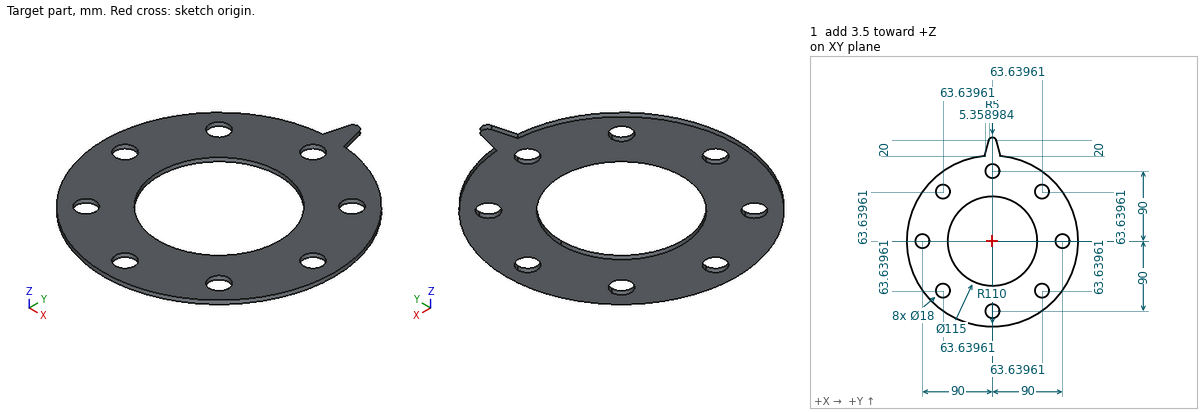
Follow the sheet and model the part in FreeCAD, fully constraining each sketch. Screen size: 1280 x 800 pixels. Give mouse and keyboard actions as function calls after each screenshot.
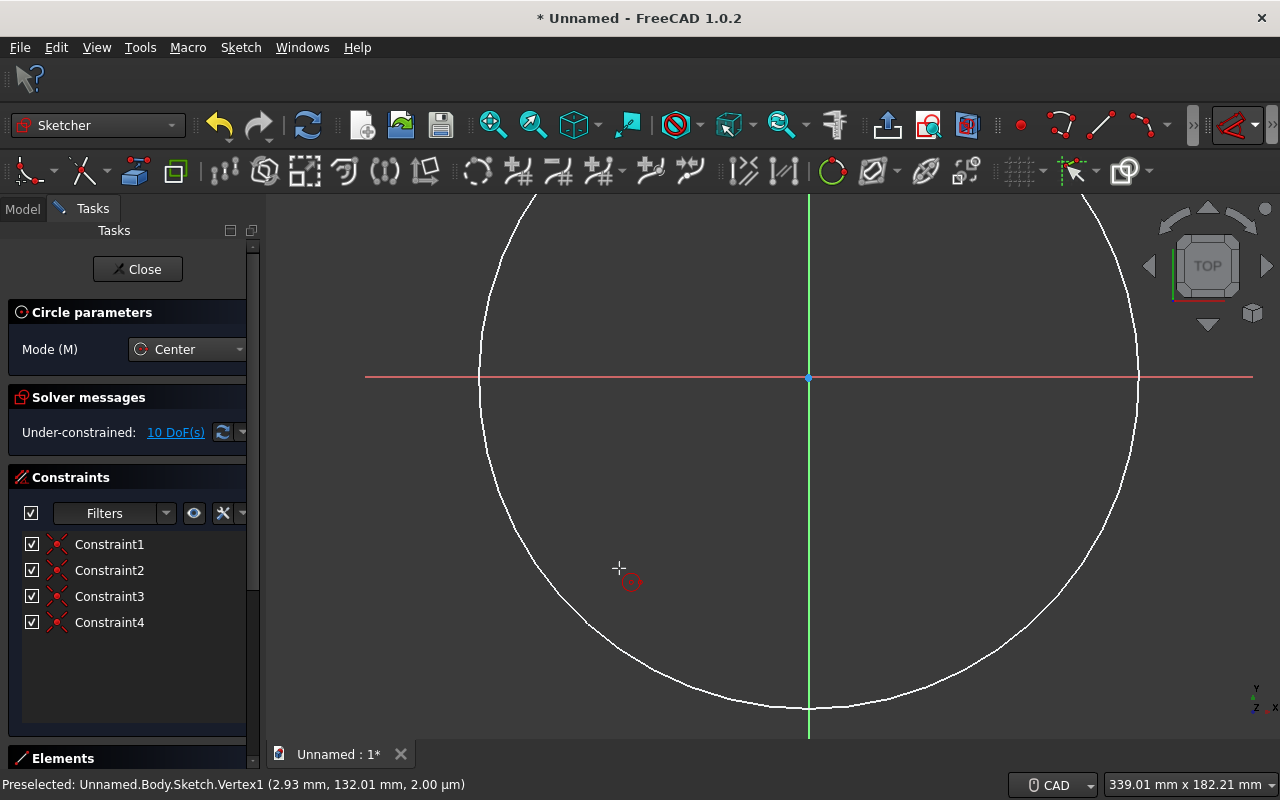
click(619, 567)
click(638, 548)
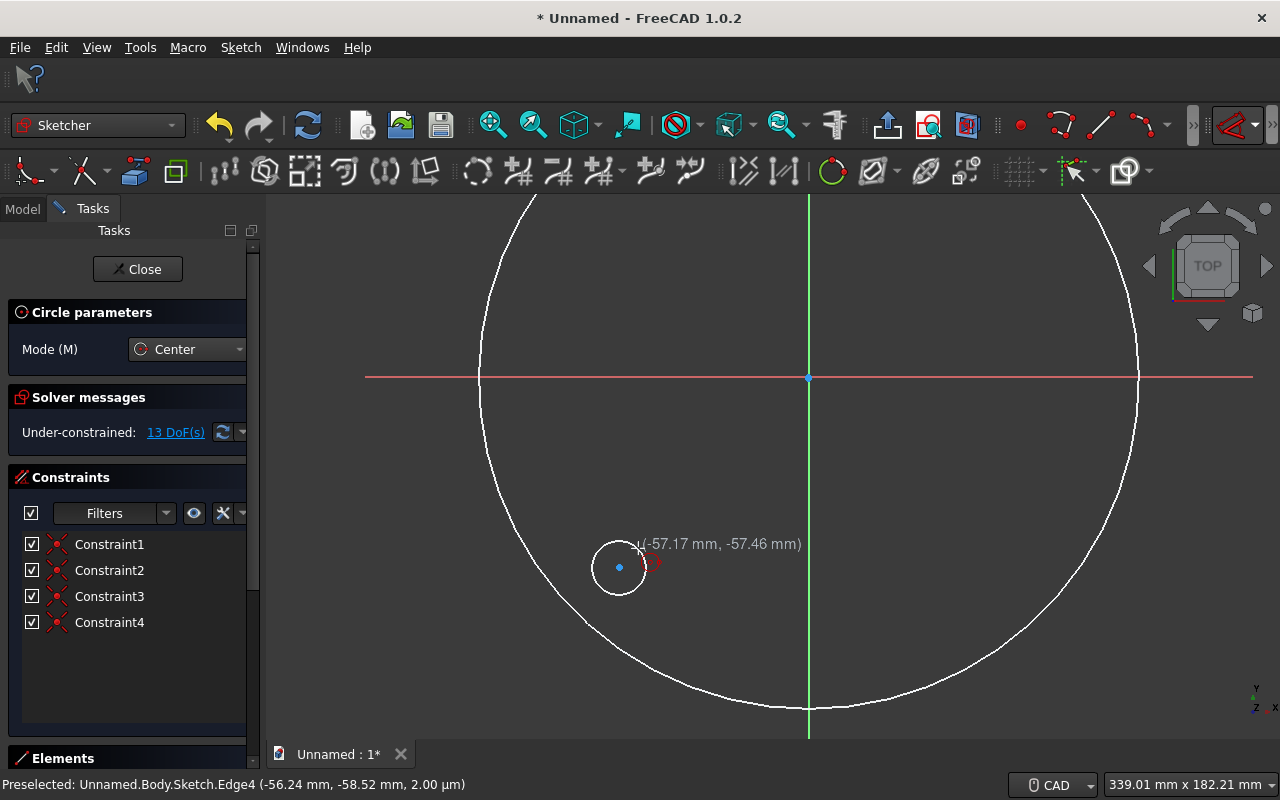
click(809, 646)
click(828, 627)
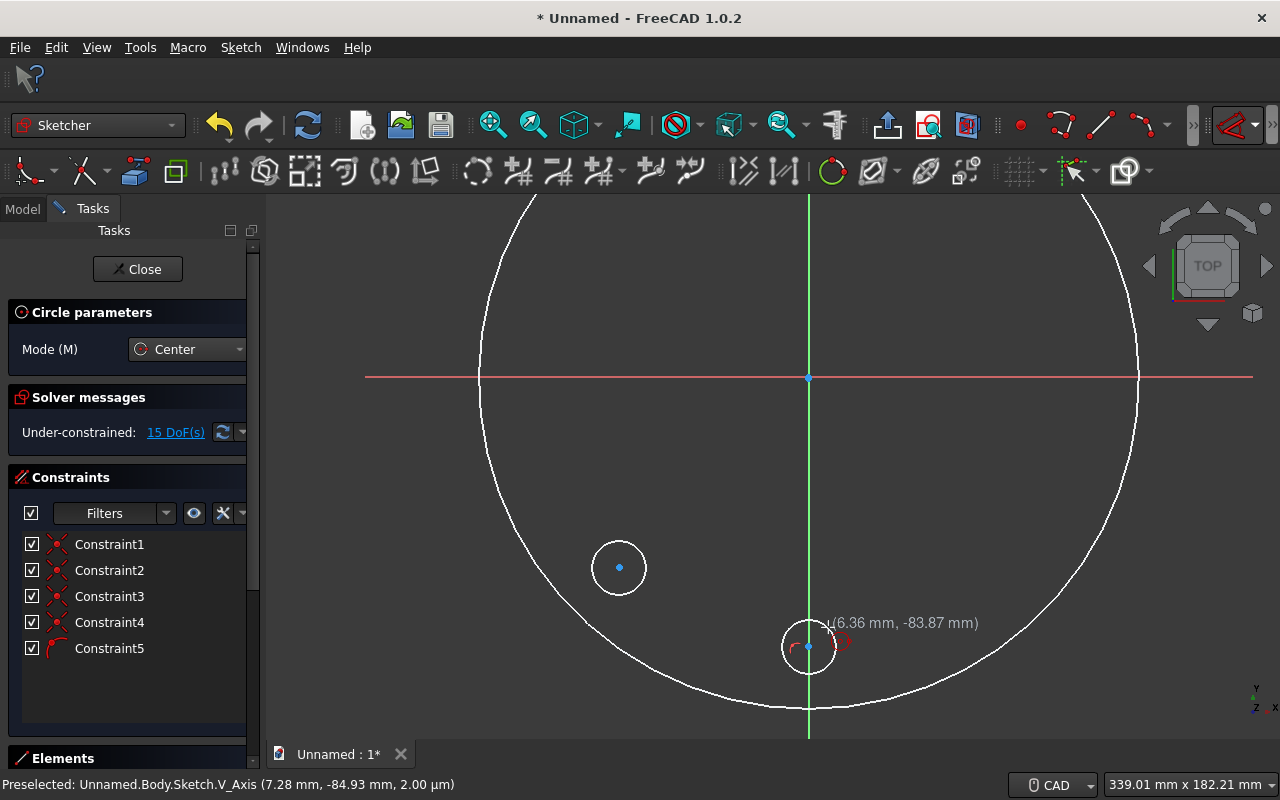
click(999, 567)
click(1018, 548)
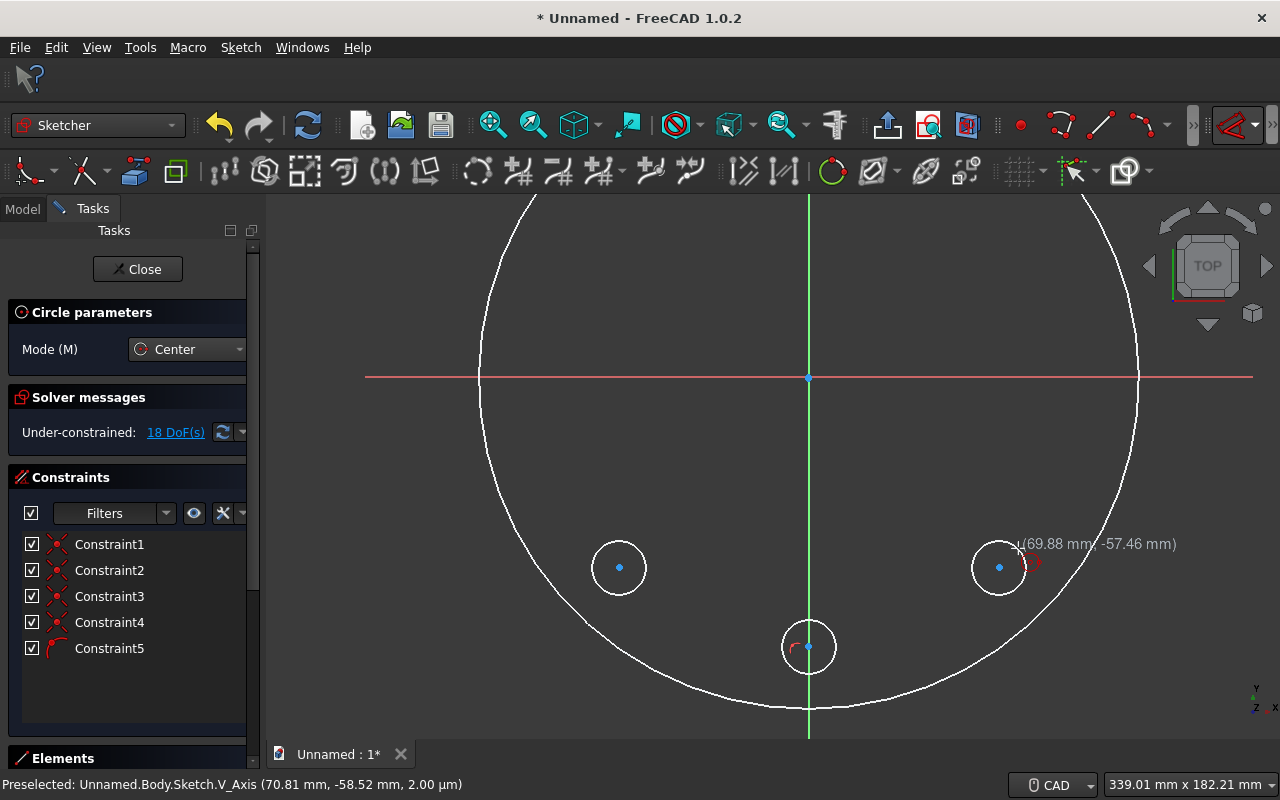
click(540, 377)
click(559, 358)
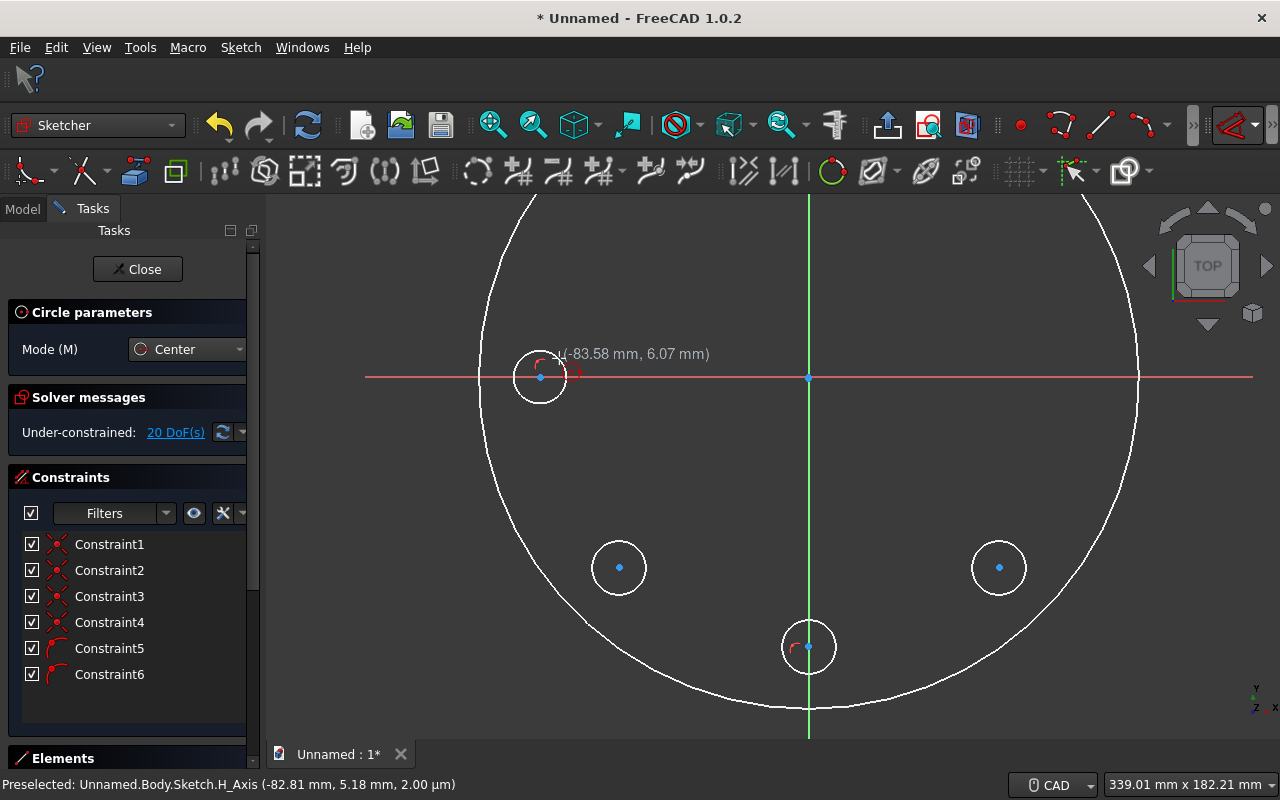
scroll(619, 568, down, 4)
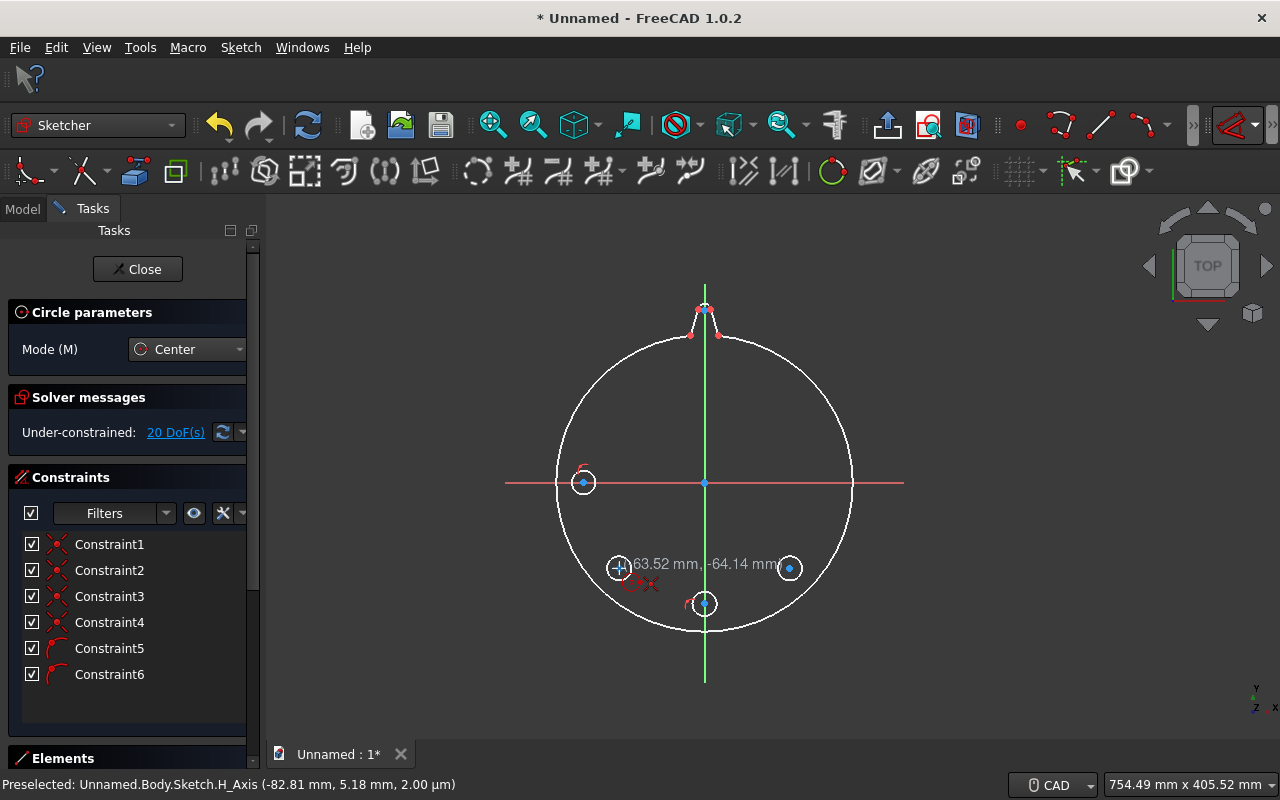
scroll(619, 397, up, 4)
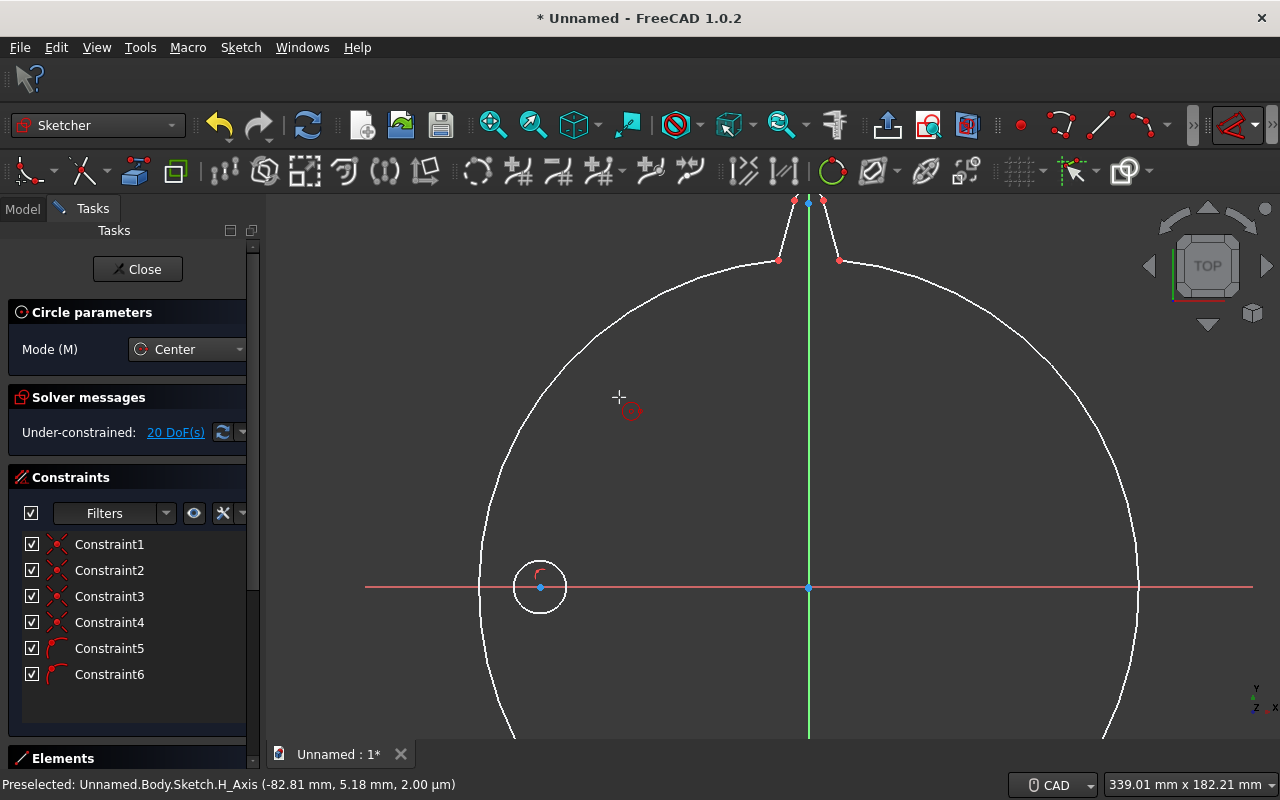
click(619, 397)
click(638, 378)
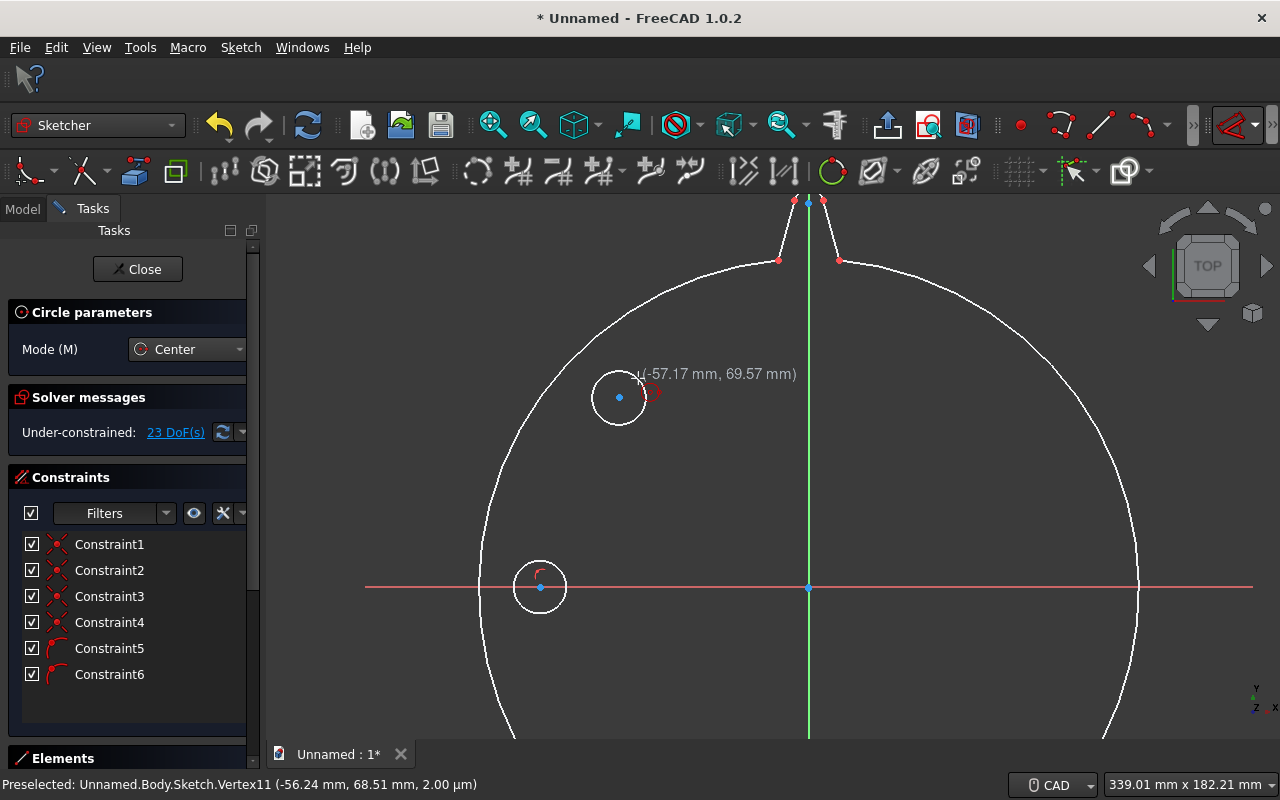
click(809, 587)
click(931, 465)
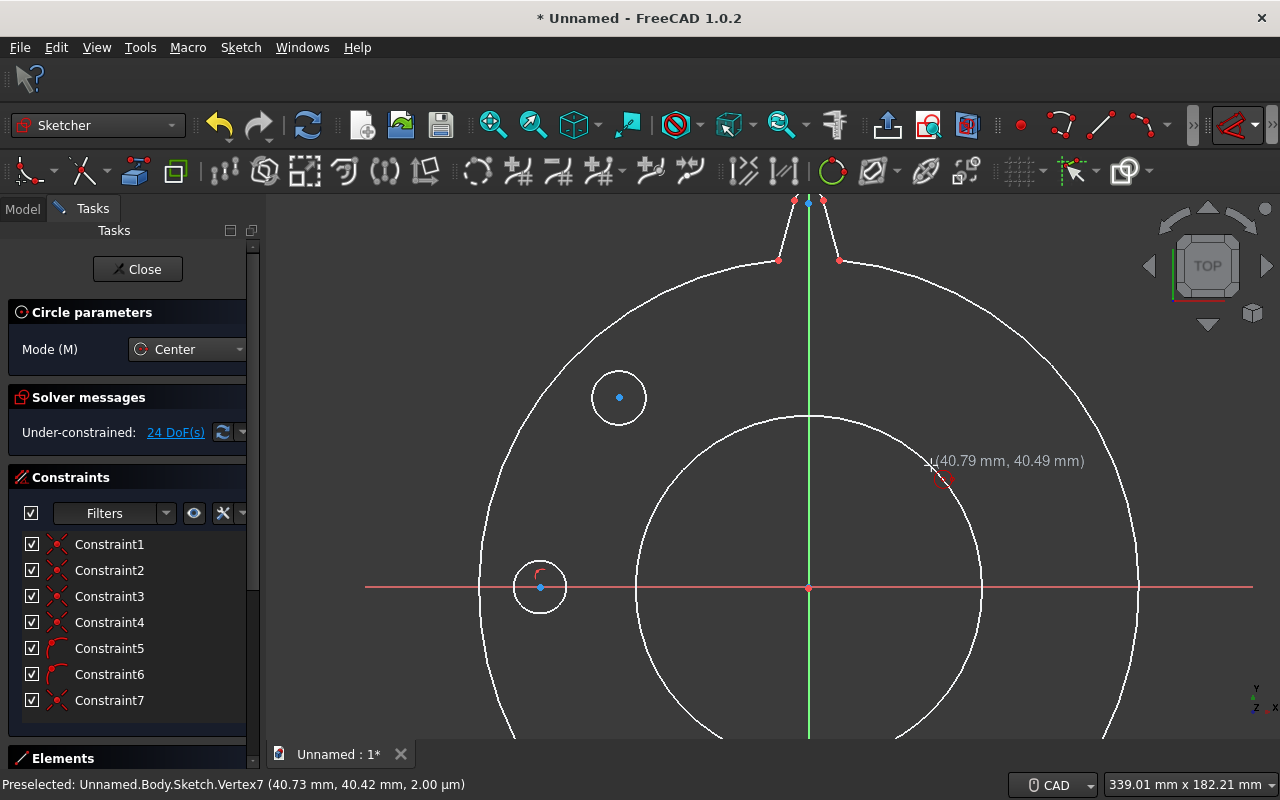
click(1078, 587)
click(1097, 568)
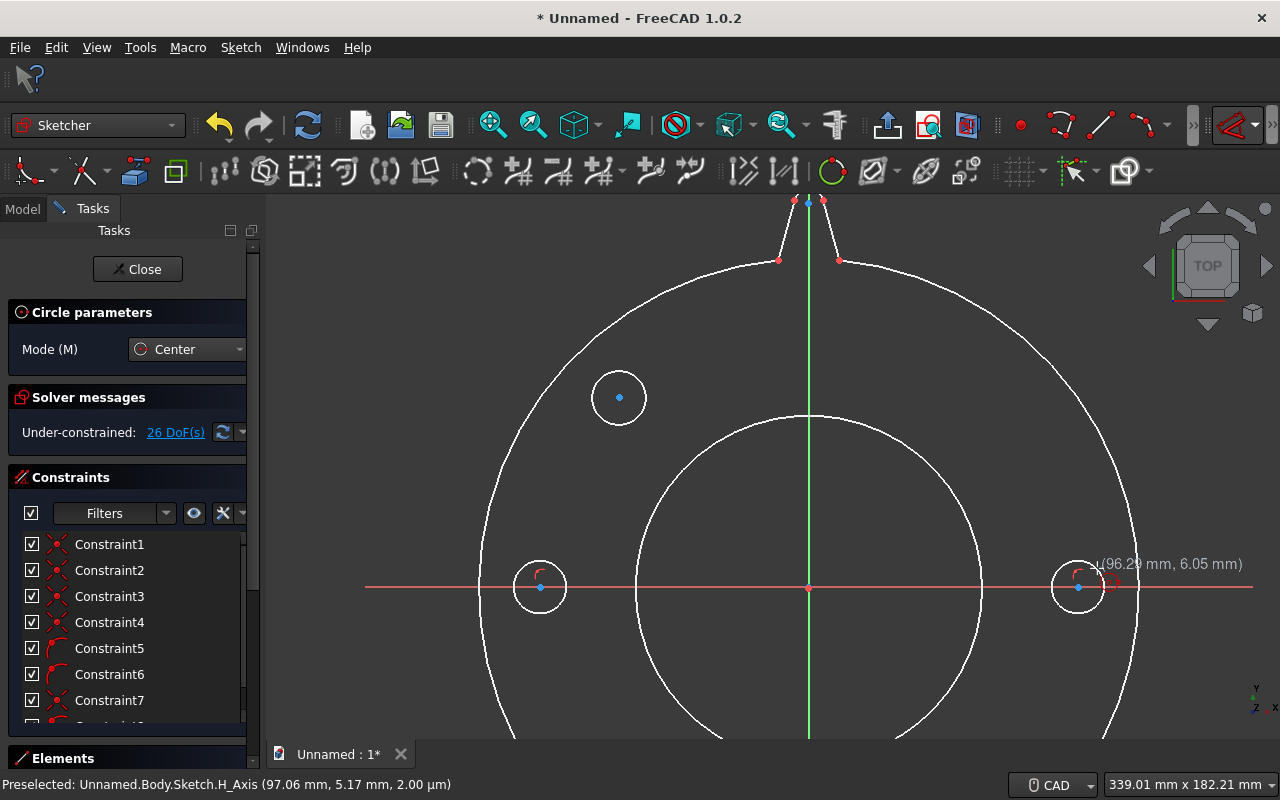
click(809, 318)
click(828, 299)